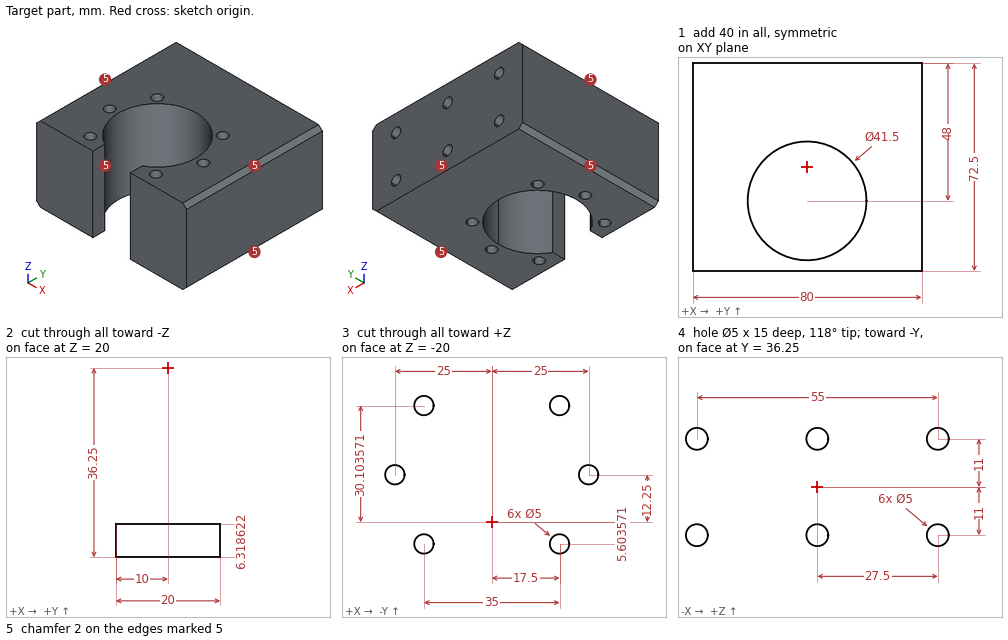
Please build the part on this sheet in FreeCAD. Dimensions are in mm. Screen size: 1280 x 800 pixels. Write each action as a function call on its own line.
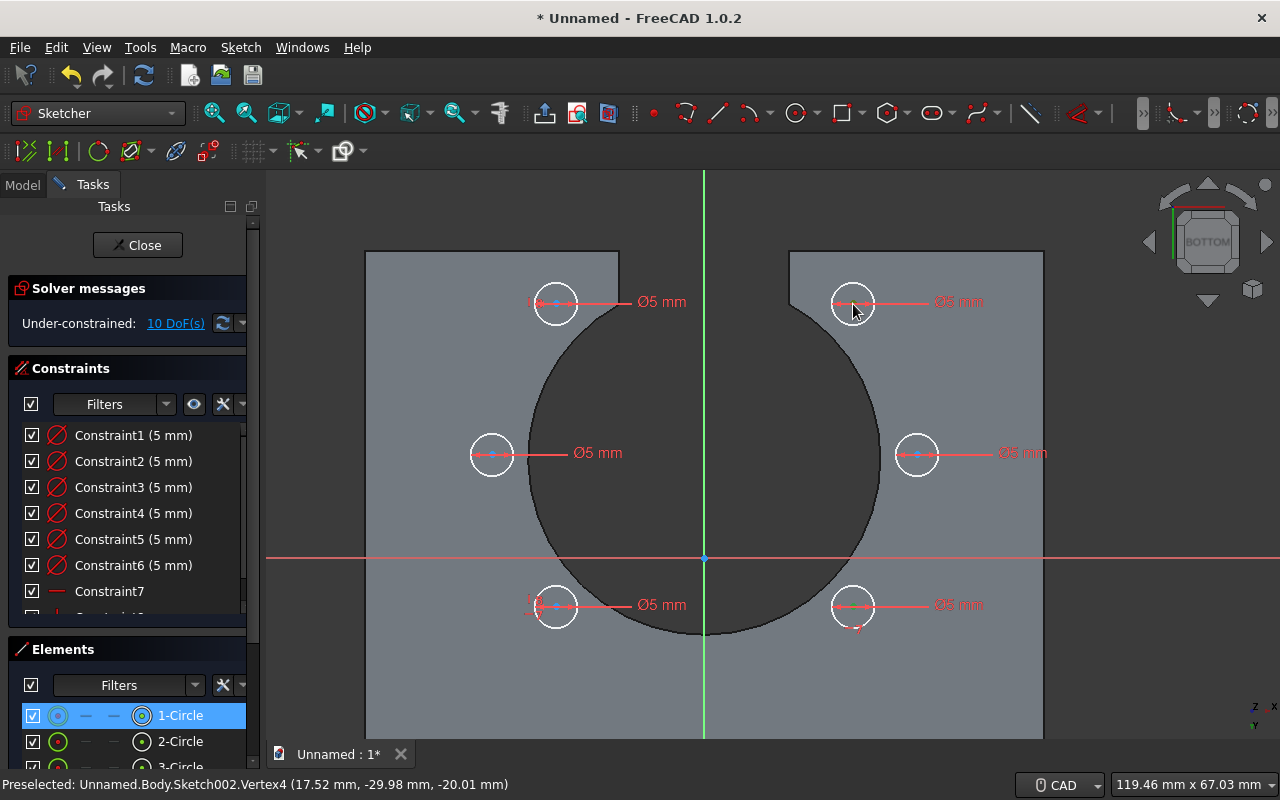
key(v)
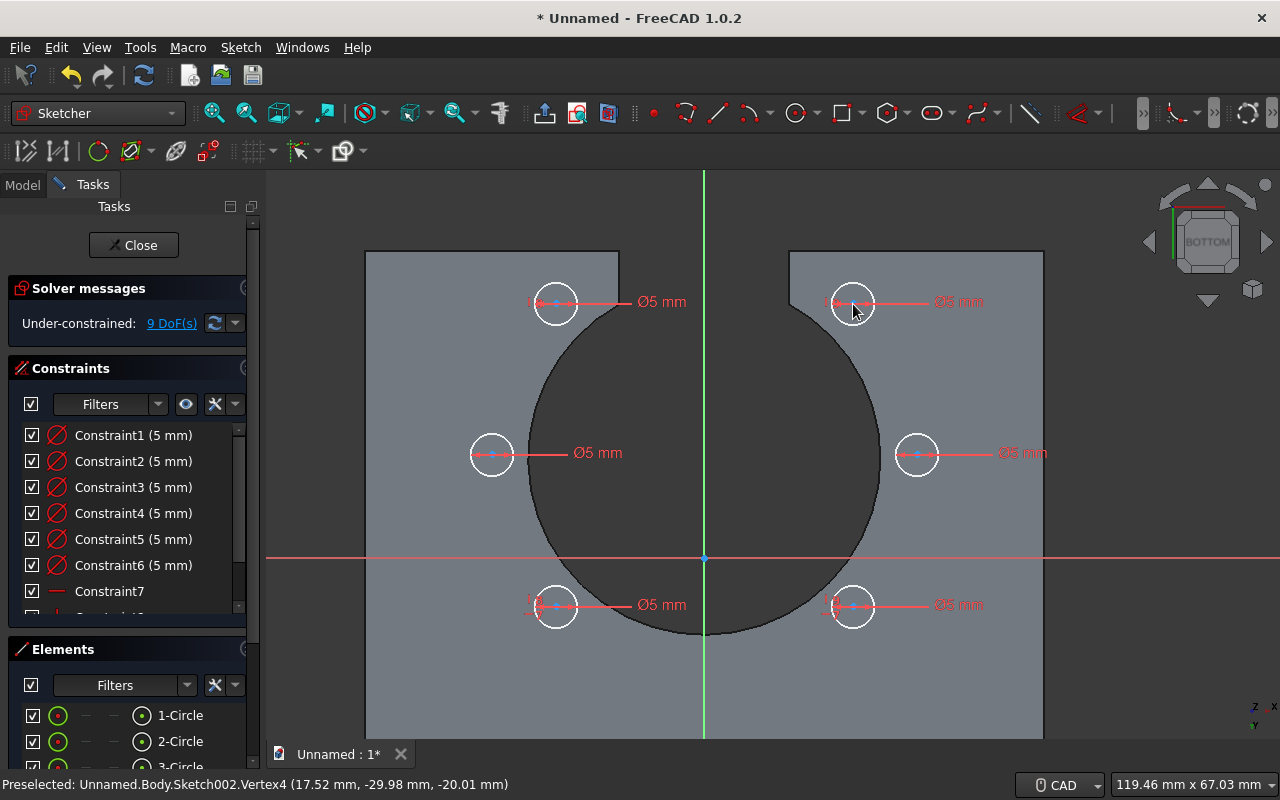
click(556, 304)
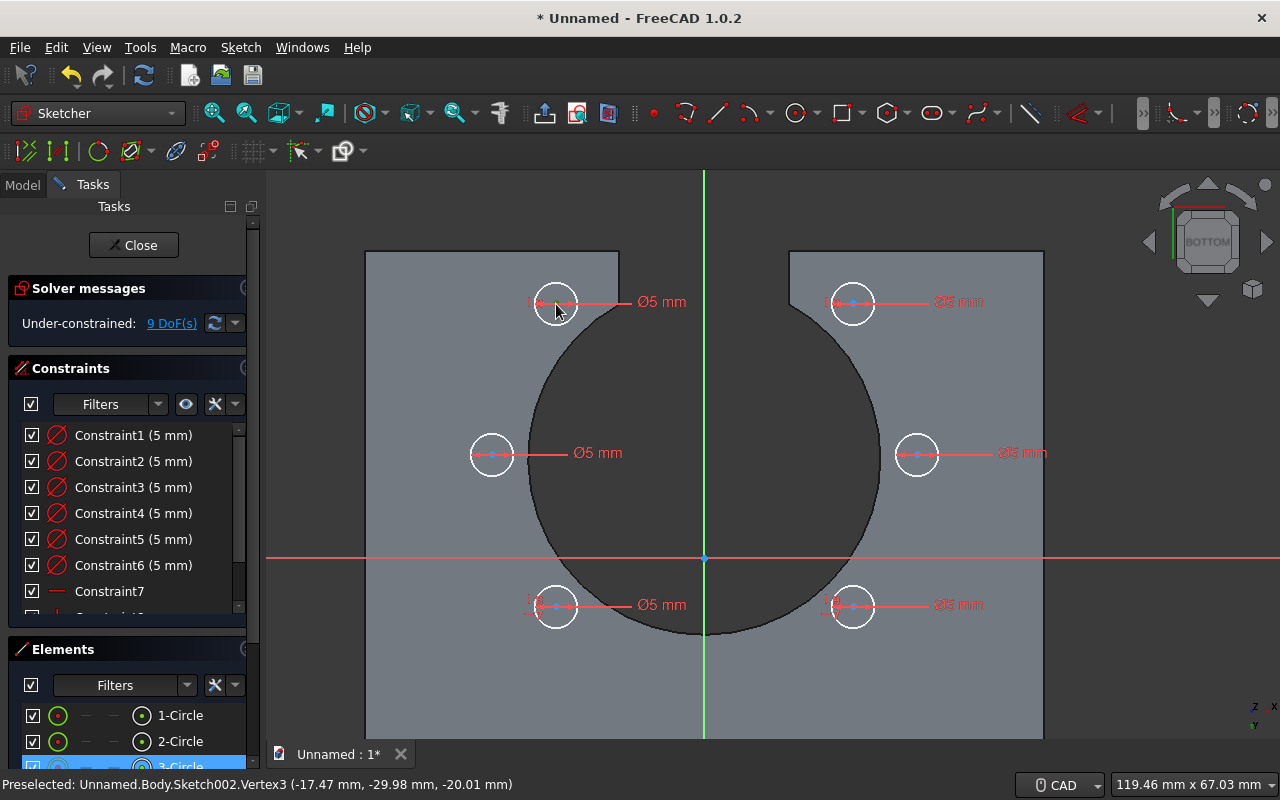
click(853, 304)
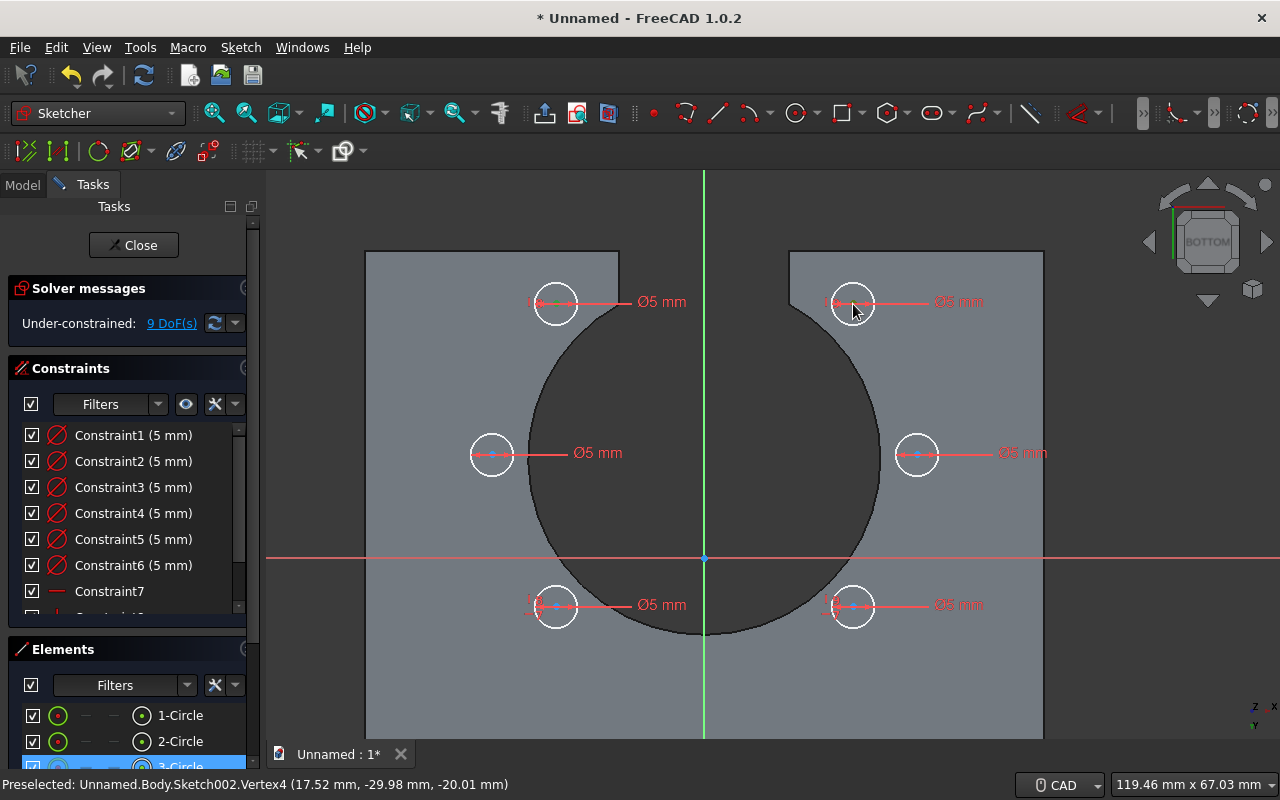
key(h)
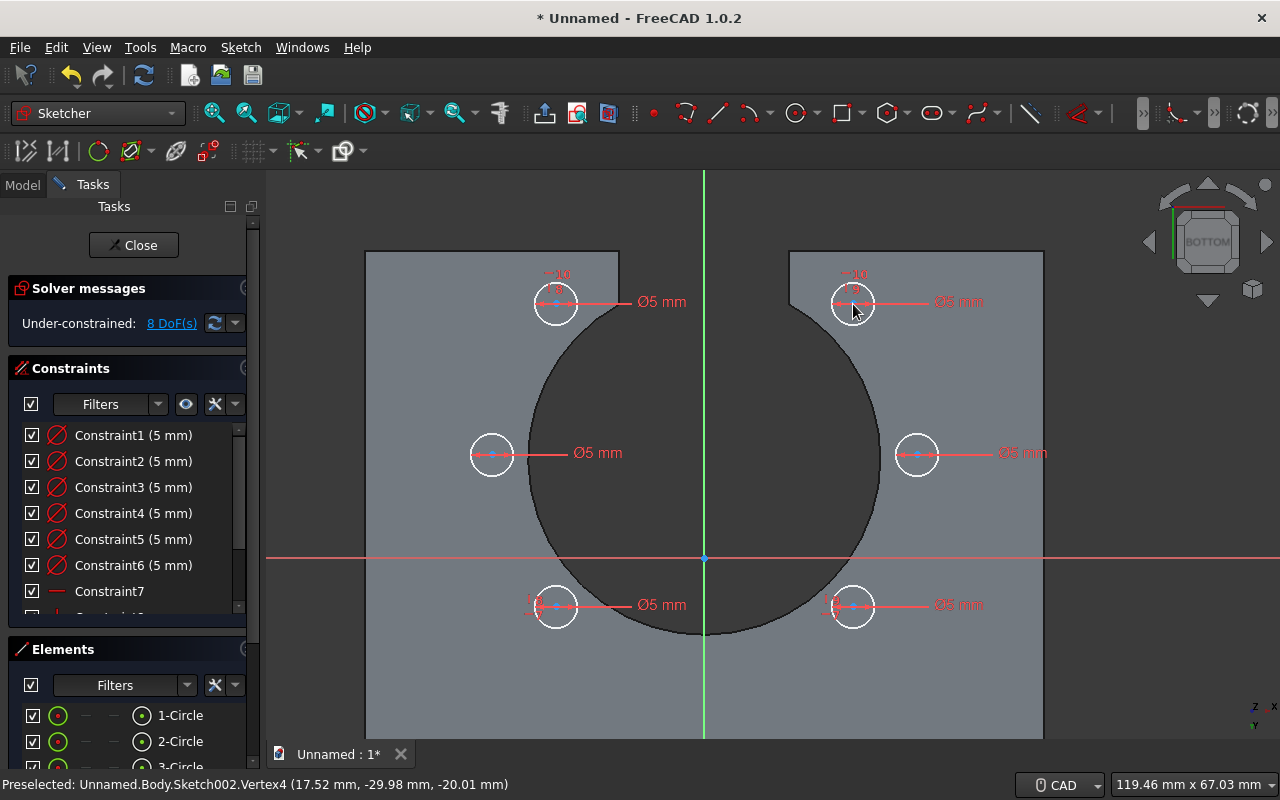
click(917, 455)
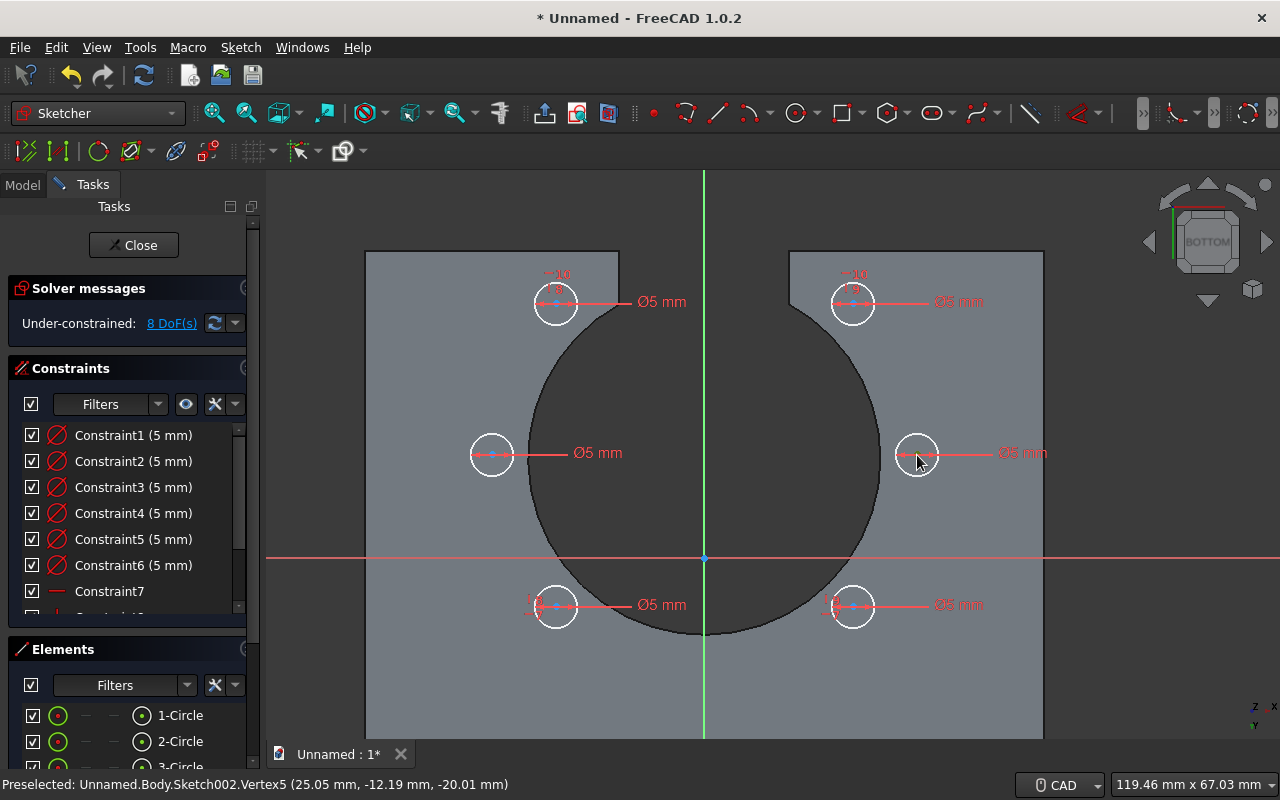
click(492, 455)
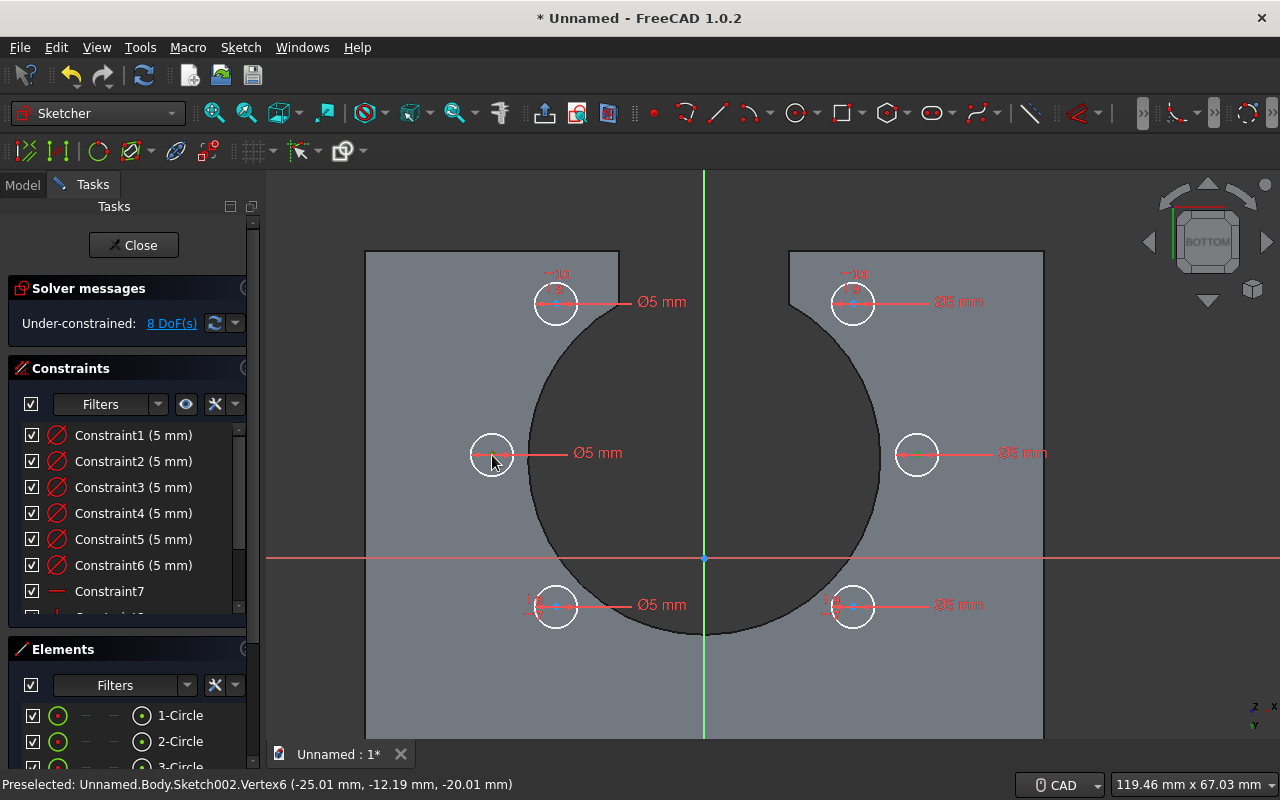
key(h)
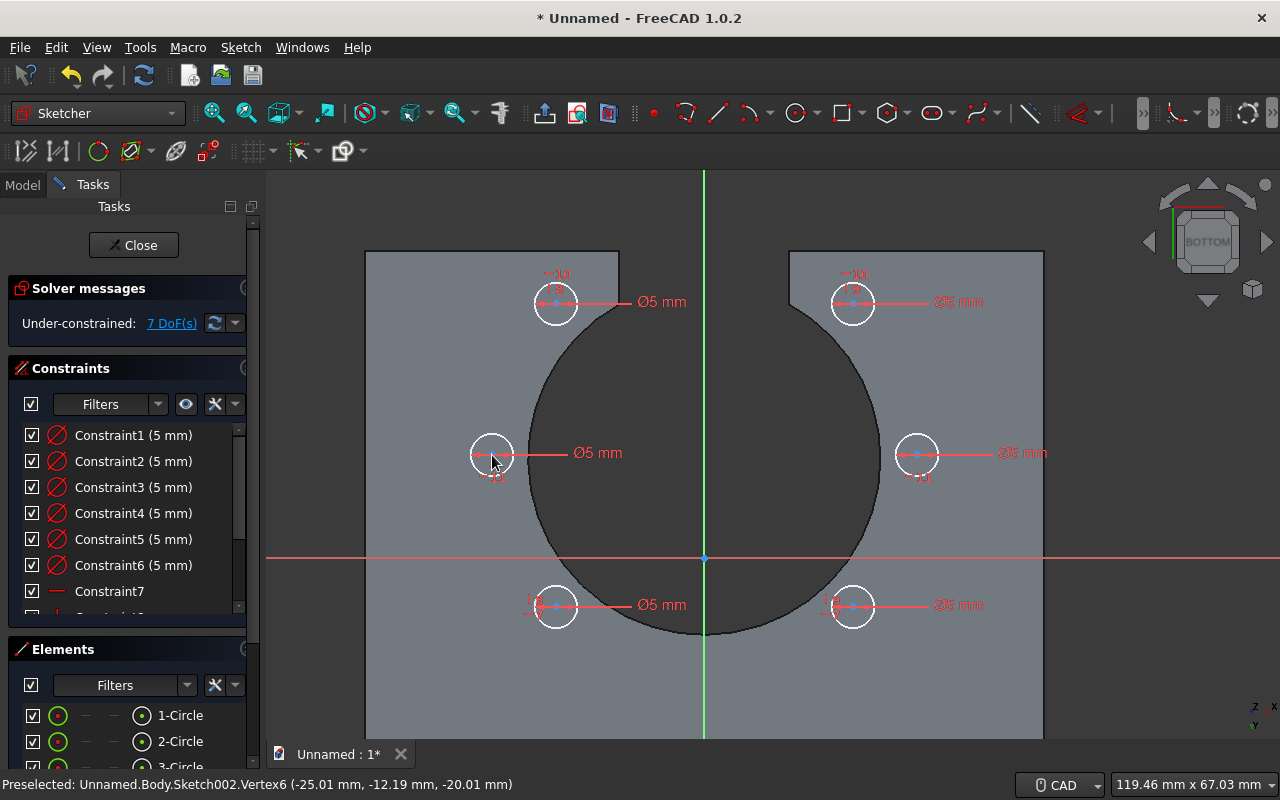
key(d)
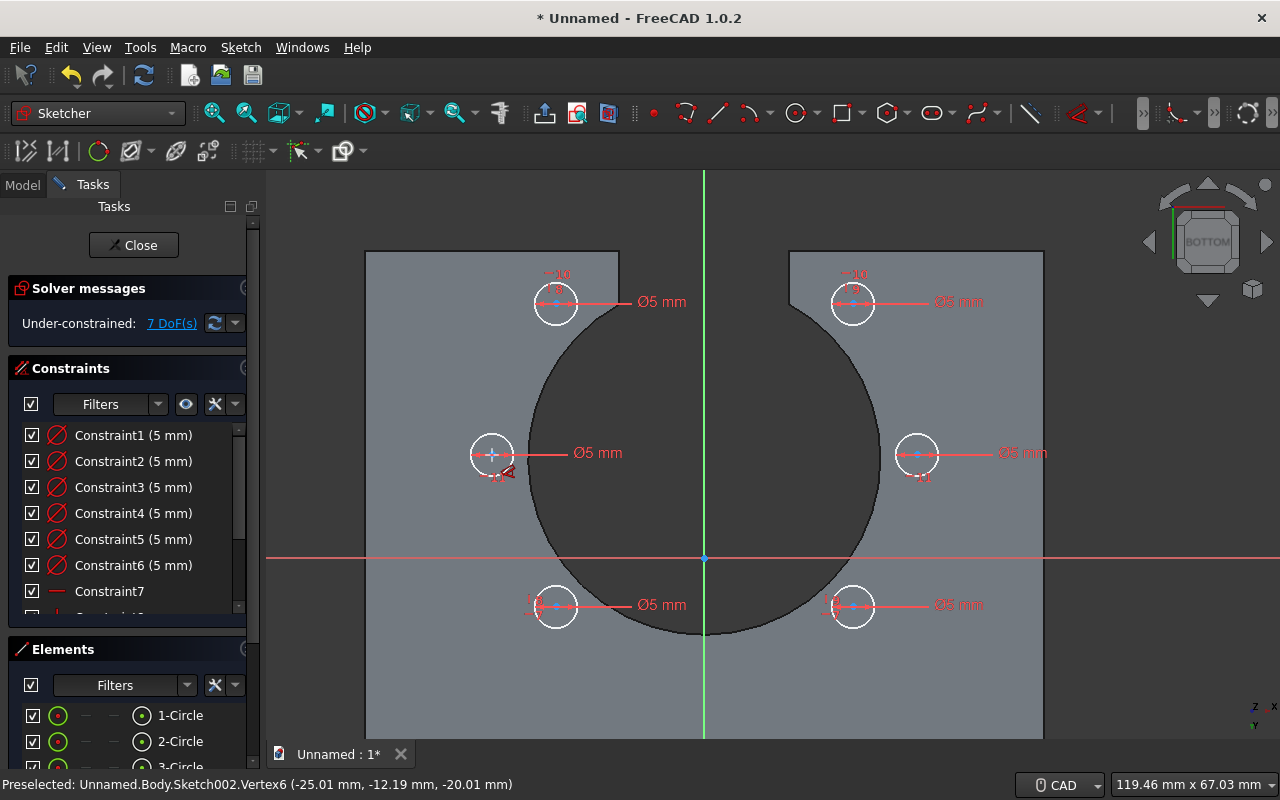
click(917, 455)
click(811, 592)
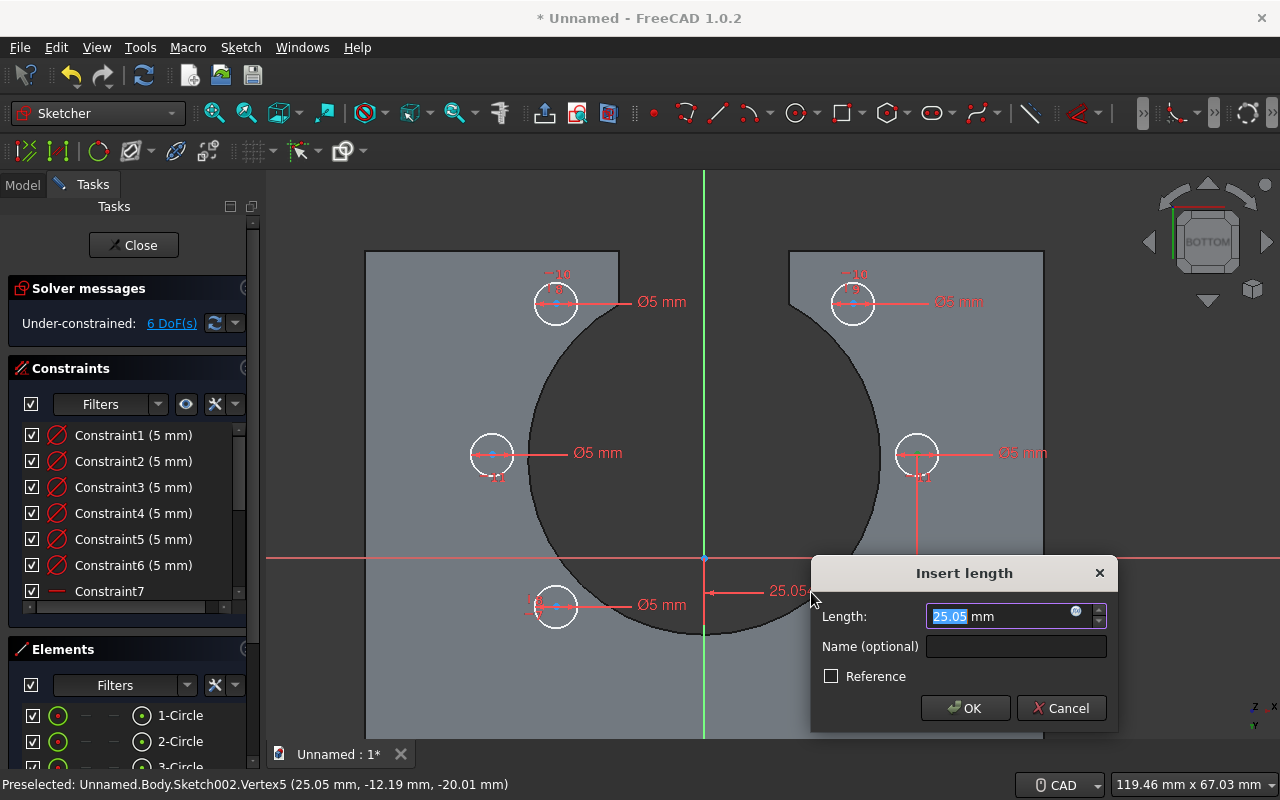
text(25)
key(Return)